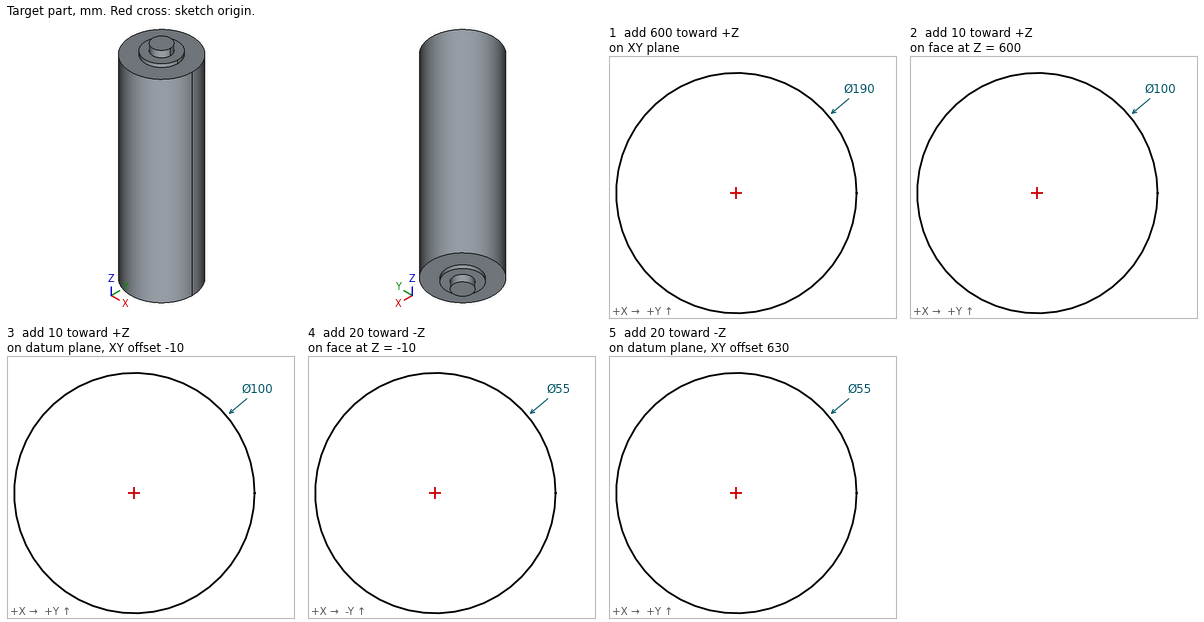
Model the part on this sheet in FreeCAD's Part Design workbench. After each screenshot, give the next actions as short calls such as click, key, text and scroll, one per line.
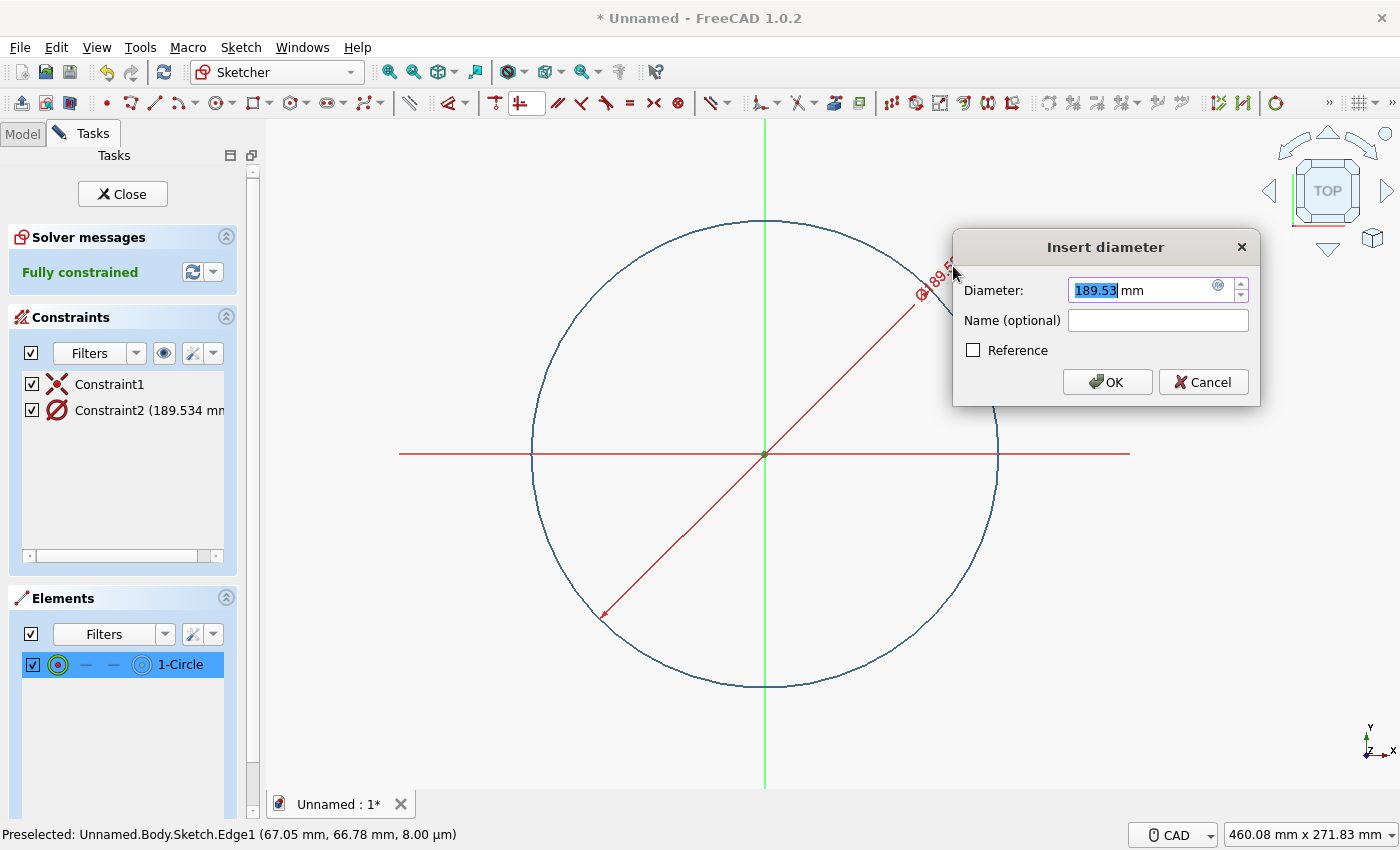
text(190)
key(Return)
key(Escape)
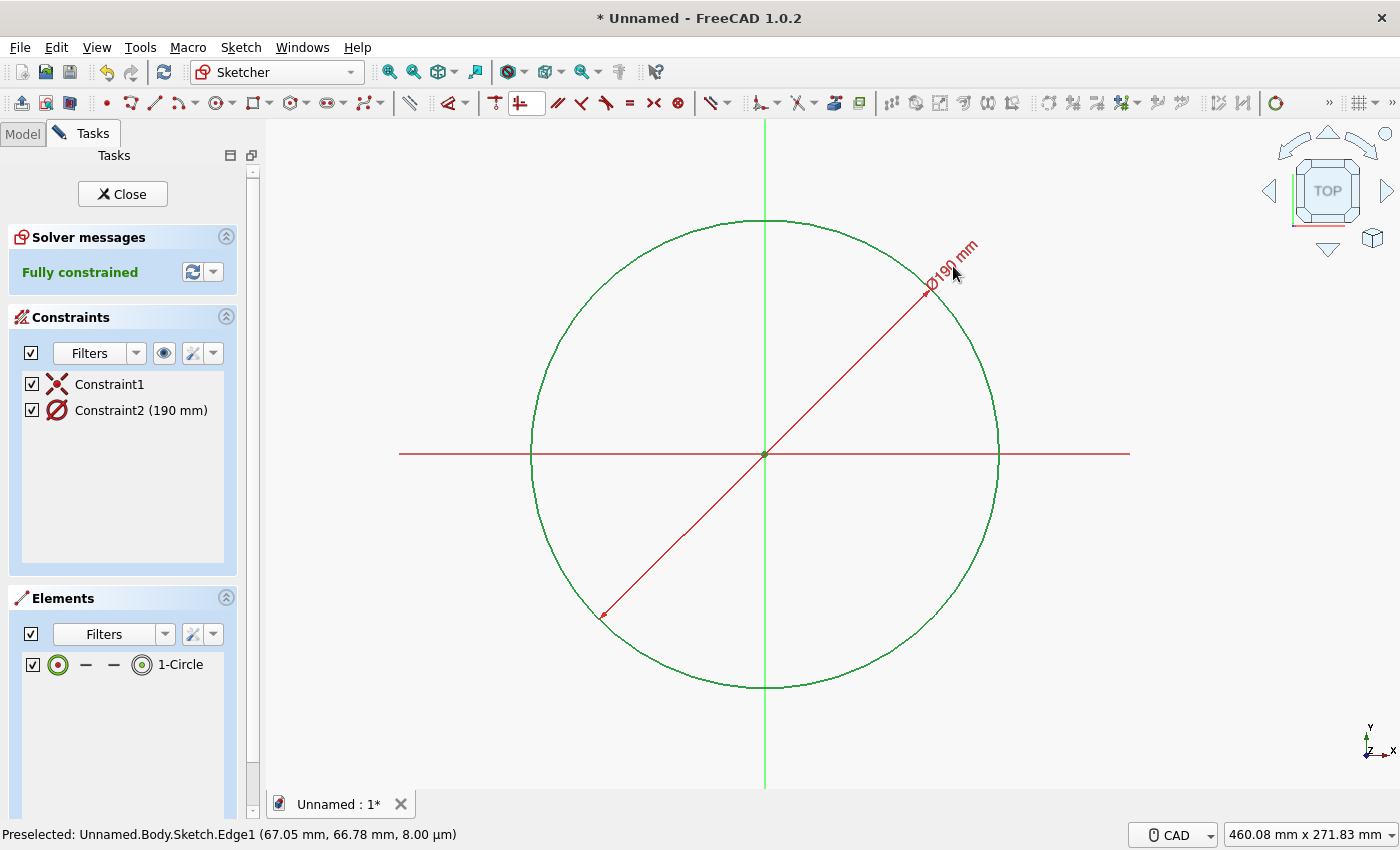
click(123, 194)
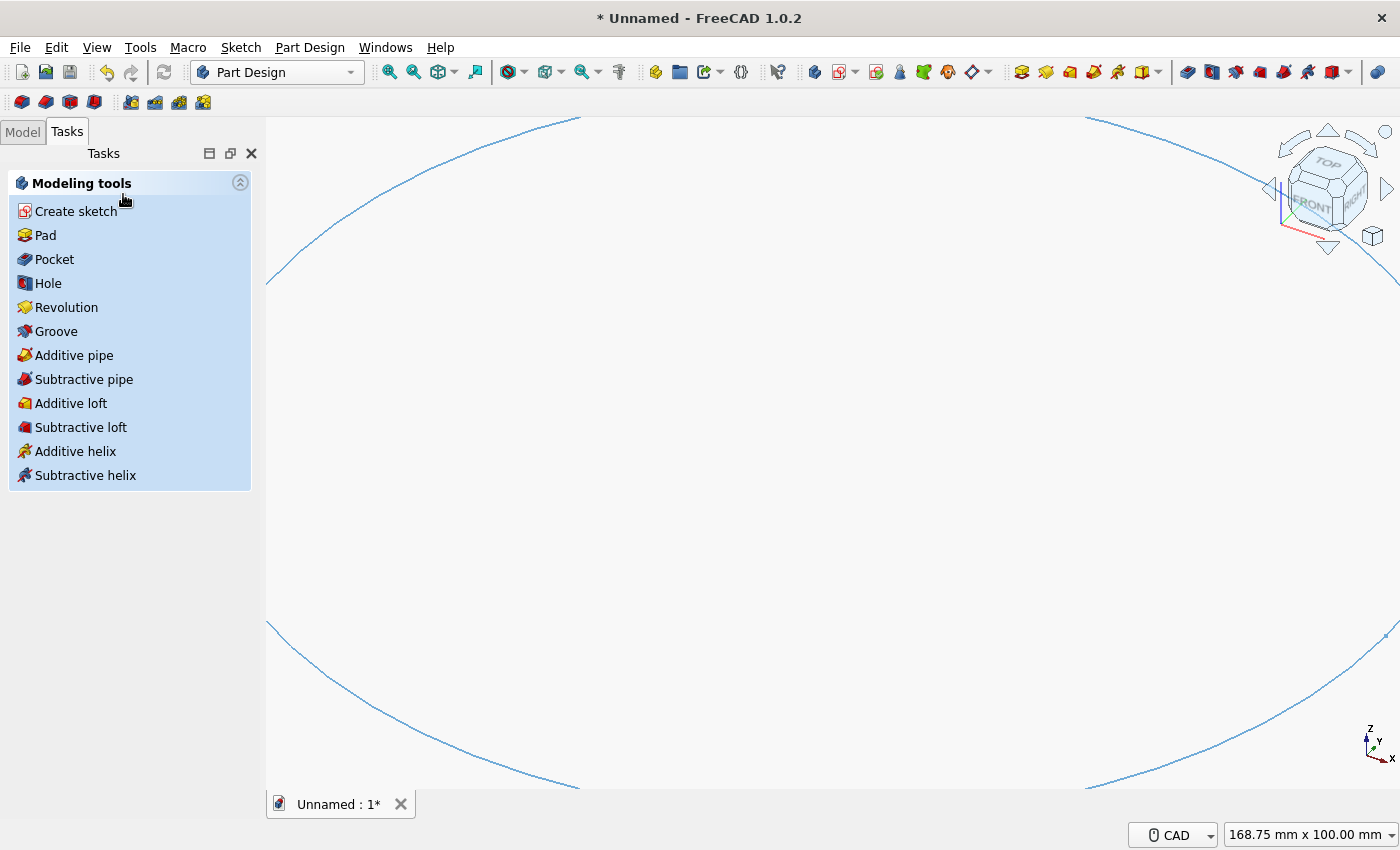
click(1022, 72)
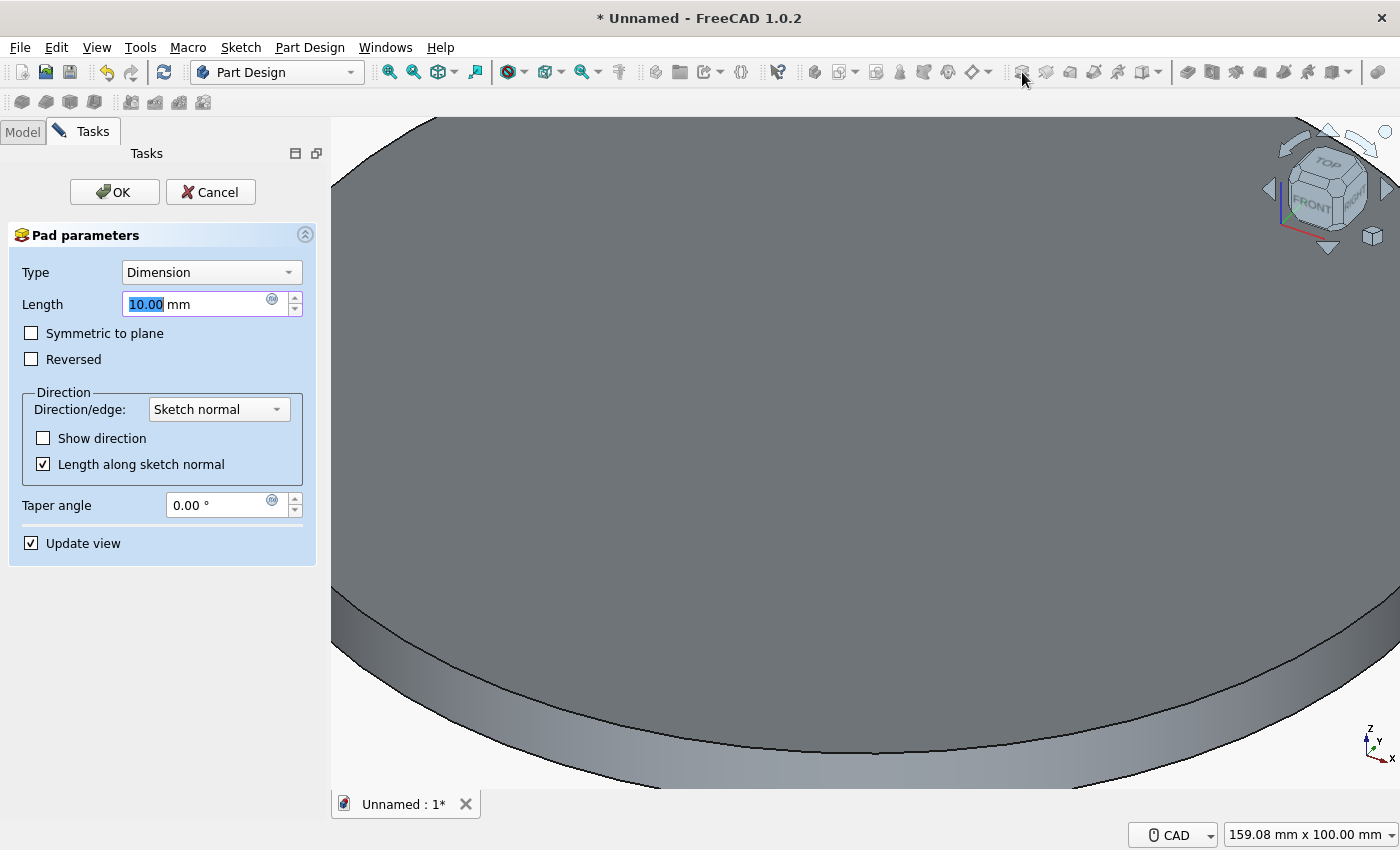
text(600)
key(Tab)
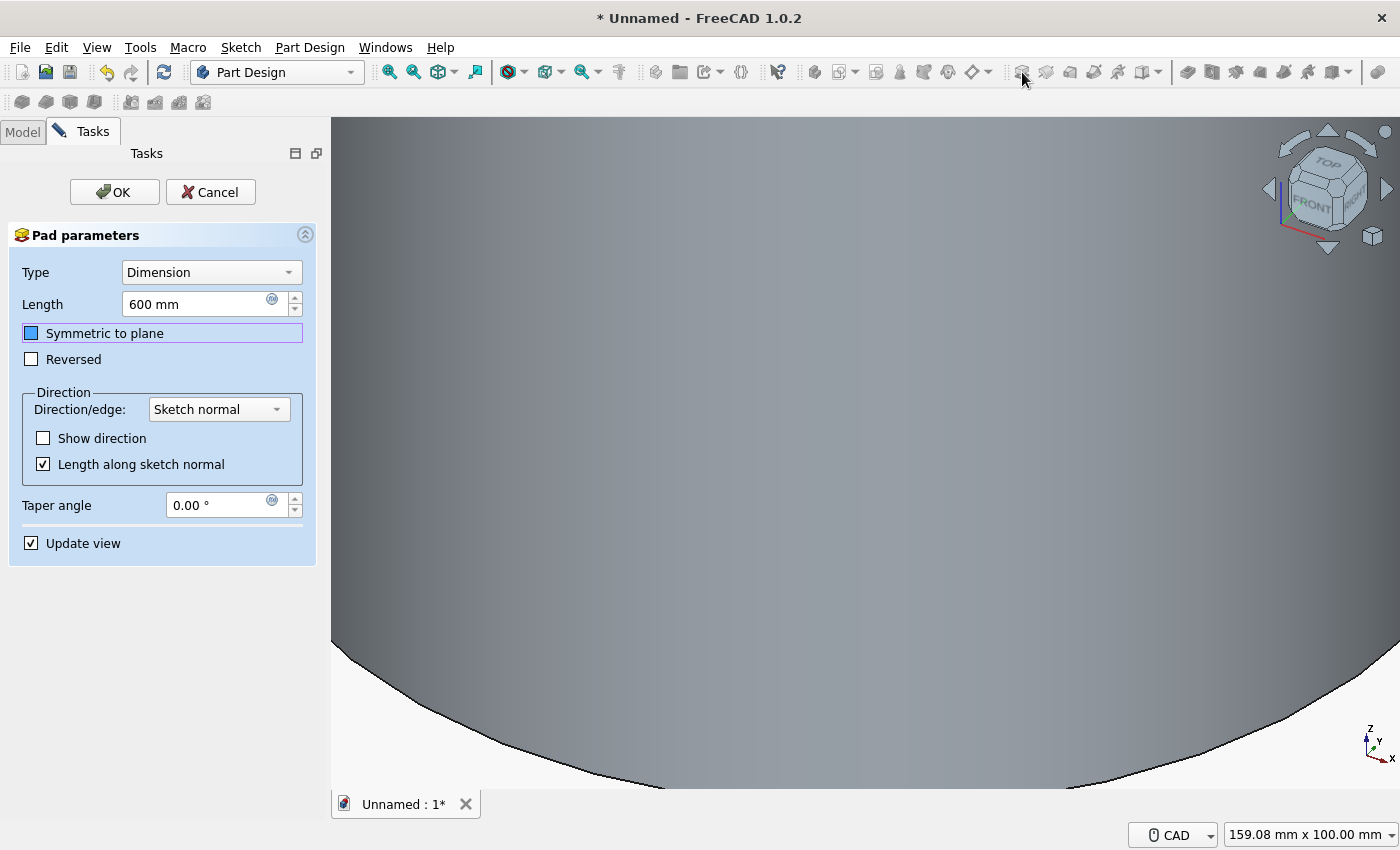
click(115, 192)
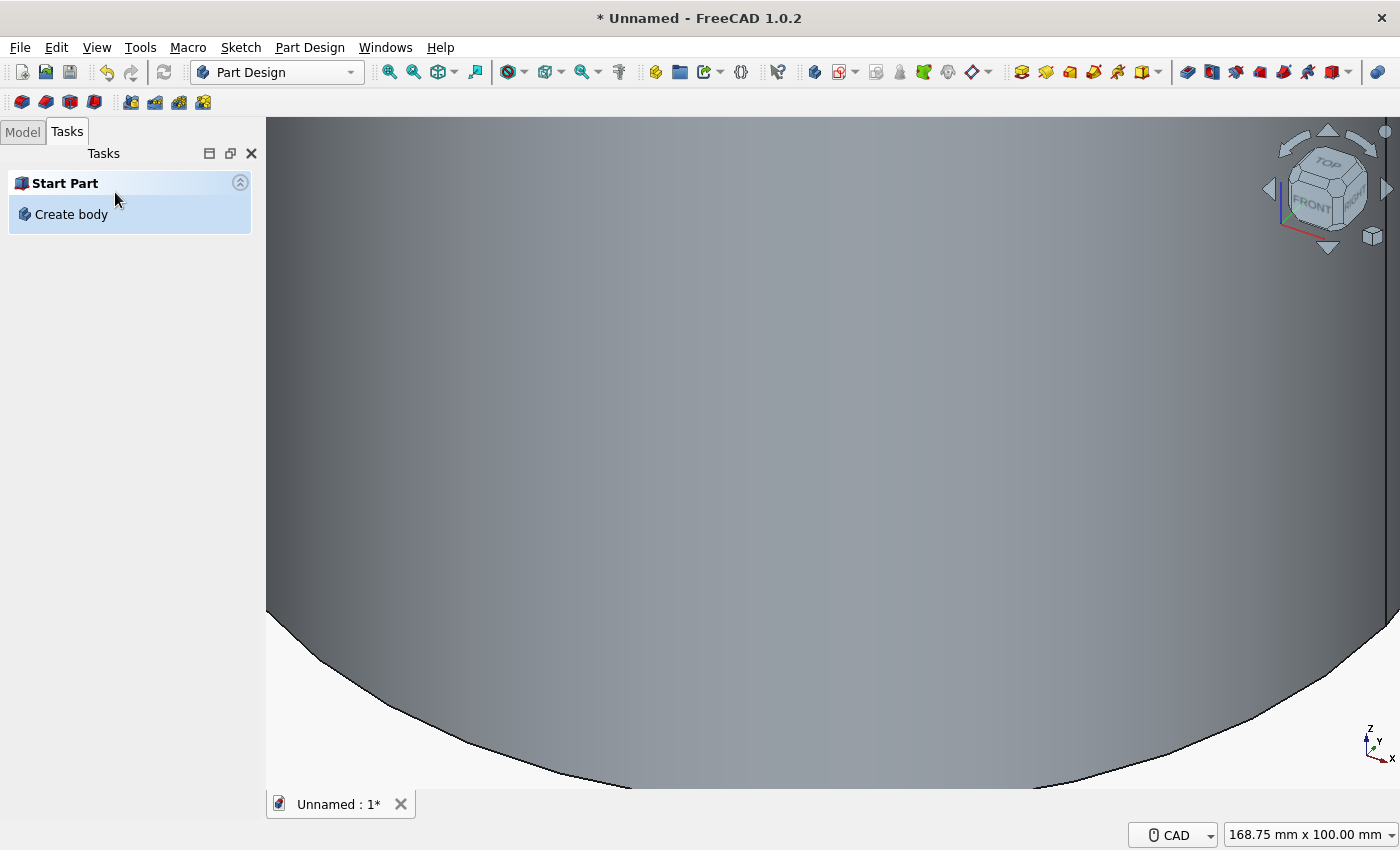
click(390, 72)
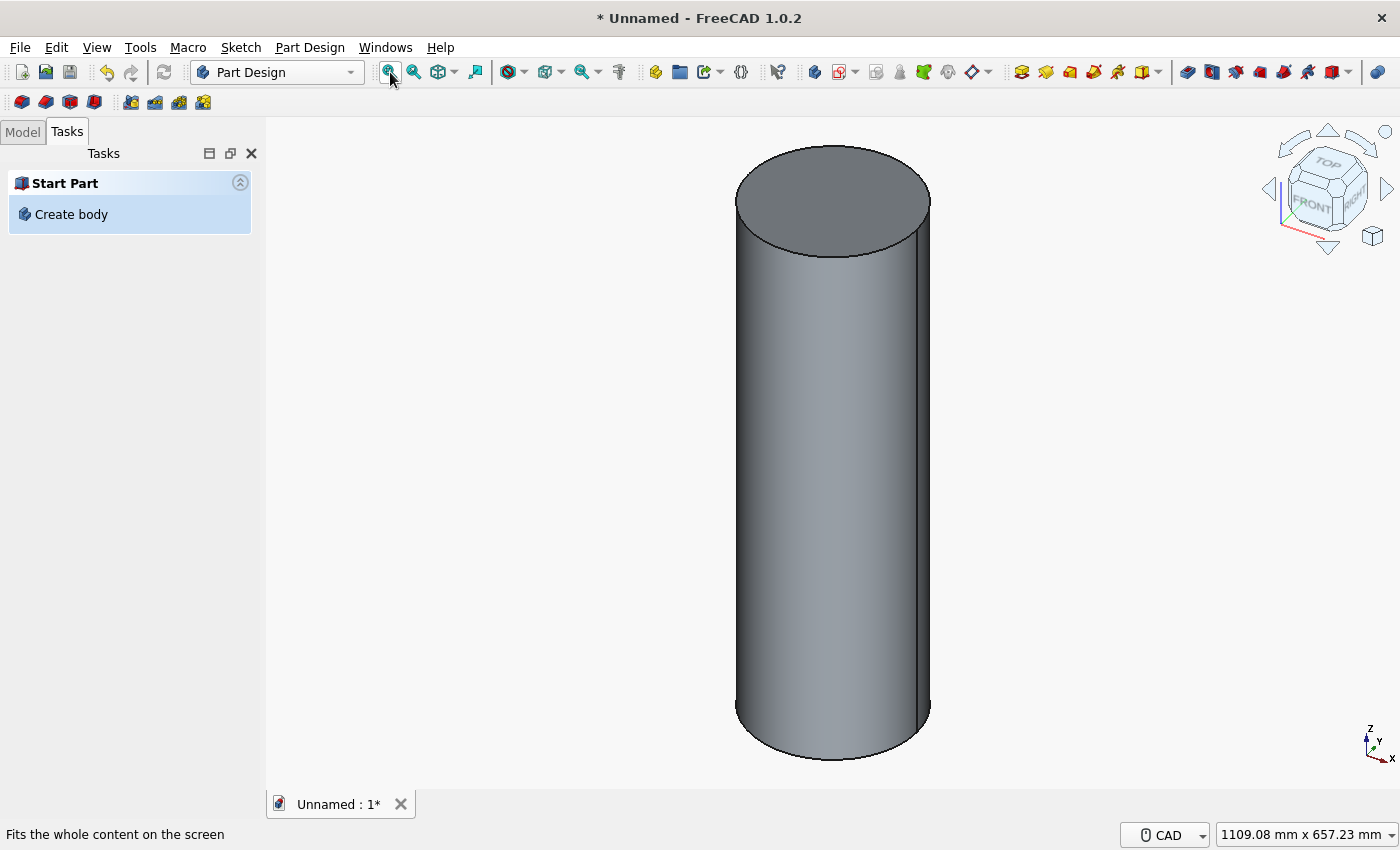
click(833, 201)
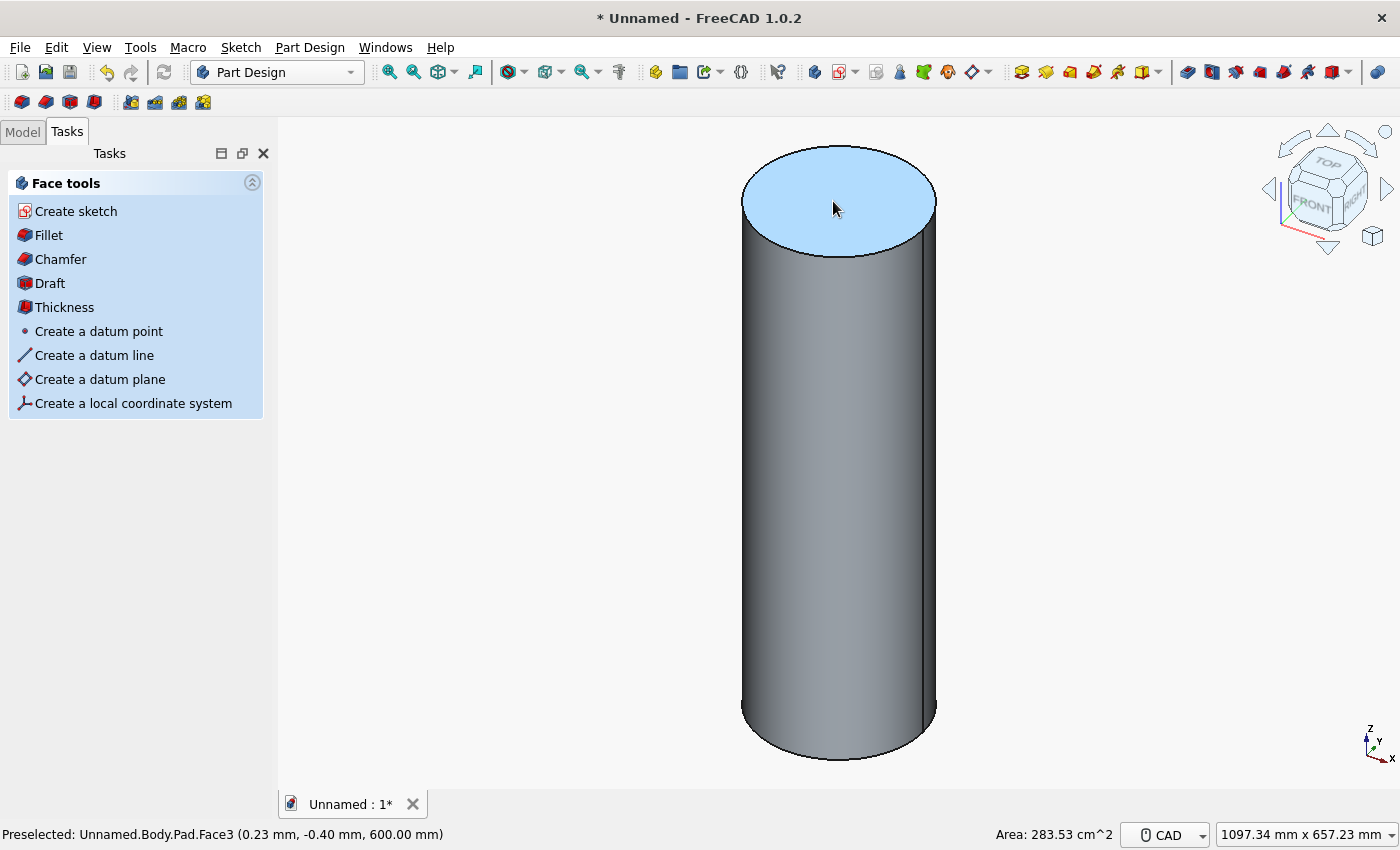
click(840, 72)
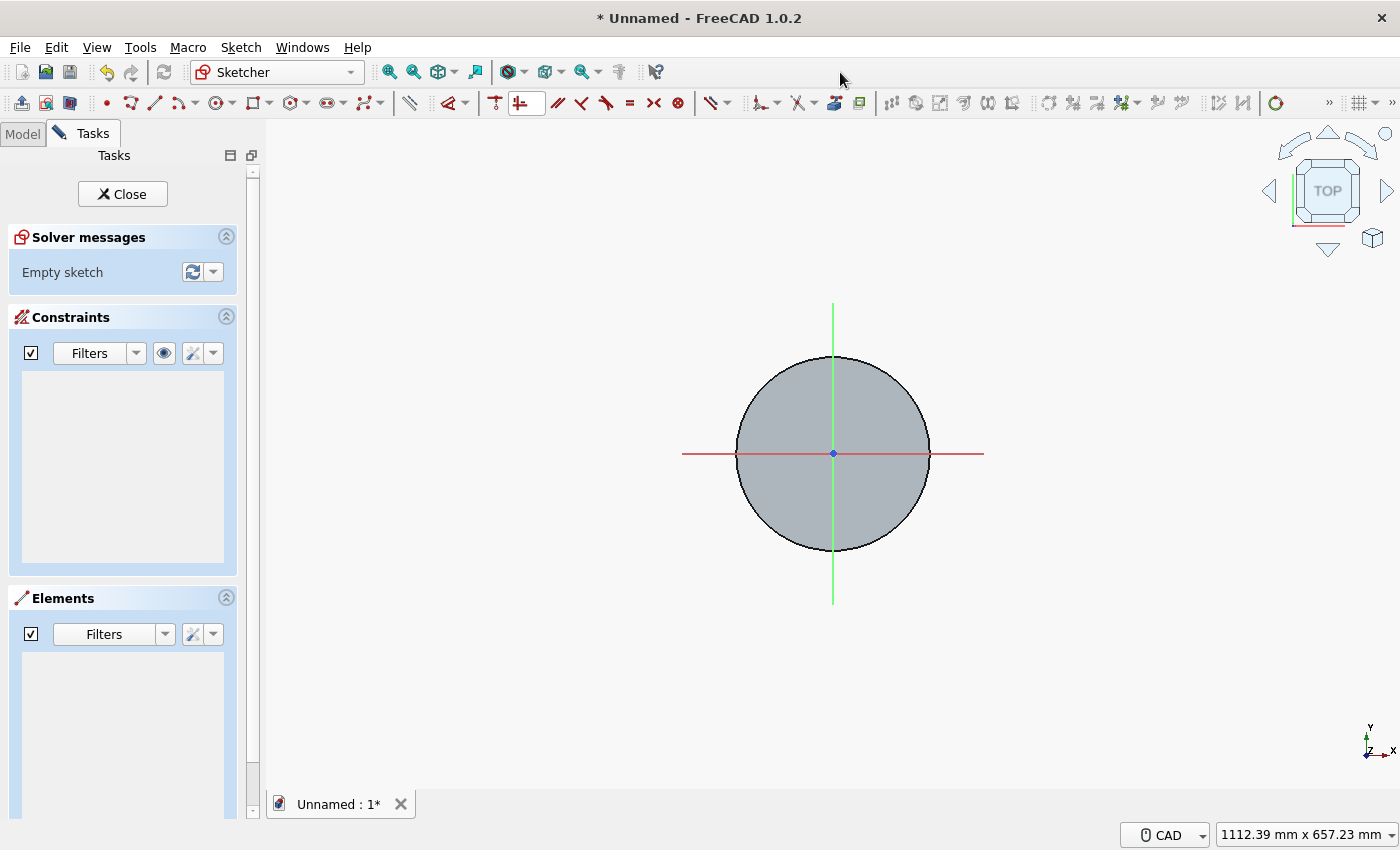
scroll(855, 454, up, 7)